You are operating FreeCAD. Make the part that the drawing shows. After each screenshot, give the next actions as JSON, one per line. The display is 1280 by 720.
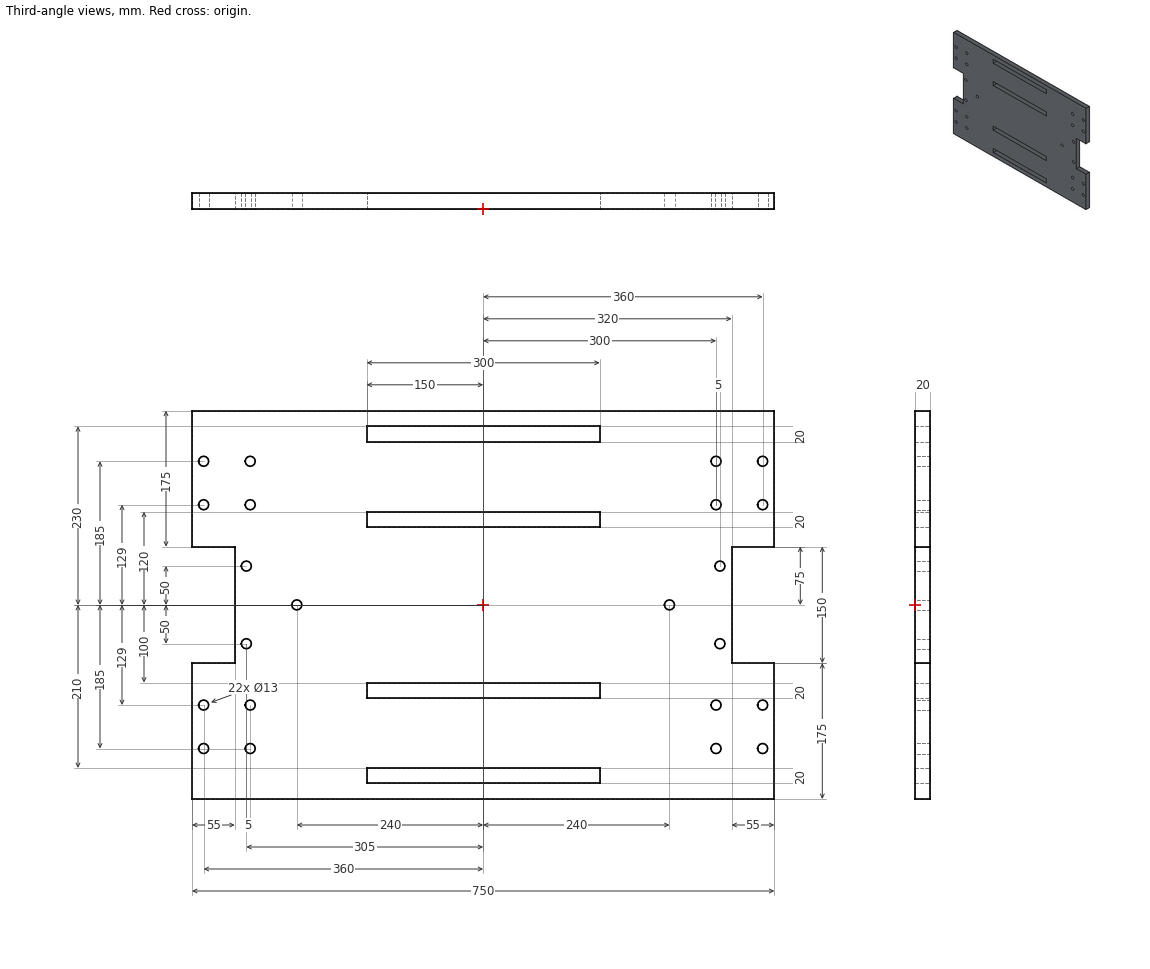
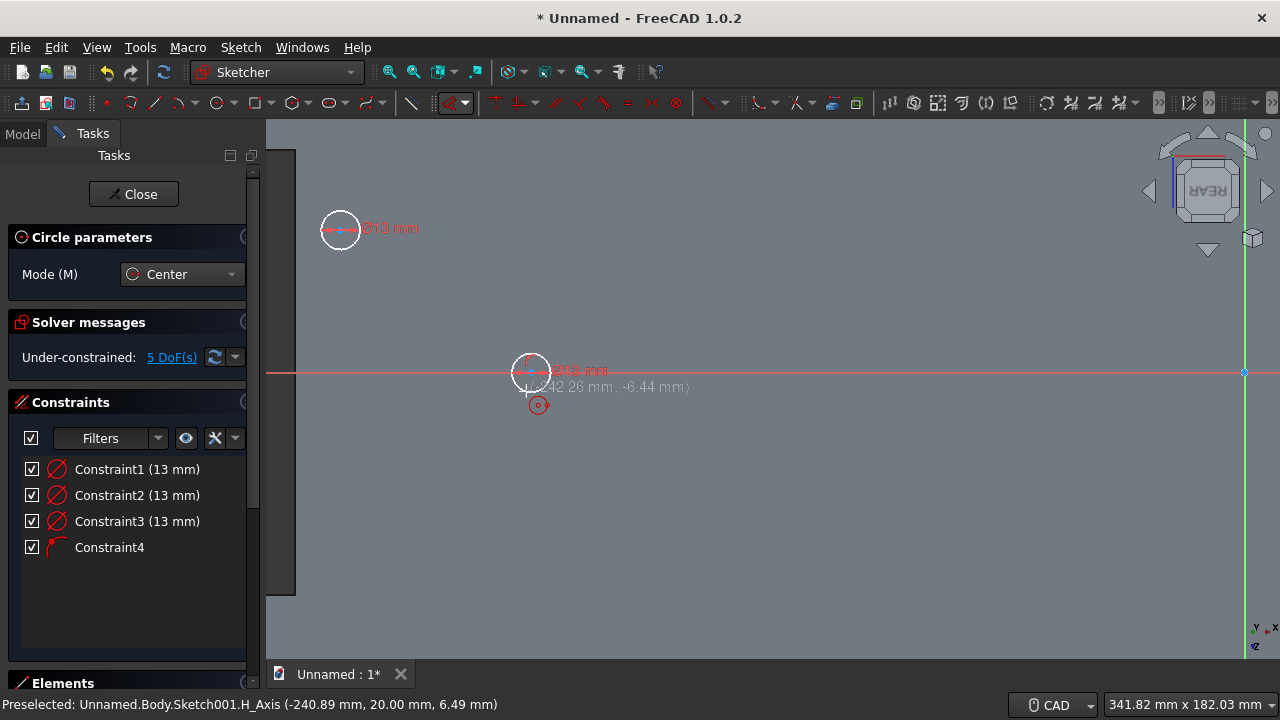
{"action": "scroll", "coordinate": [528, 394], "scroll_direction": "down", "scroll_amount": 7}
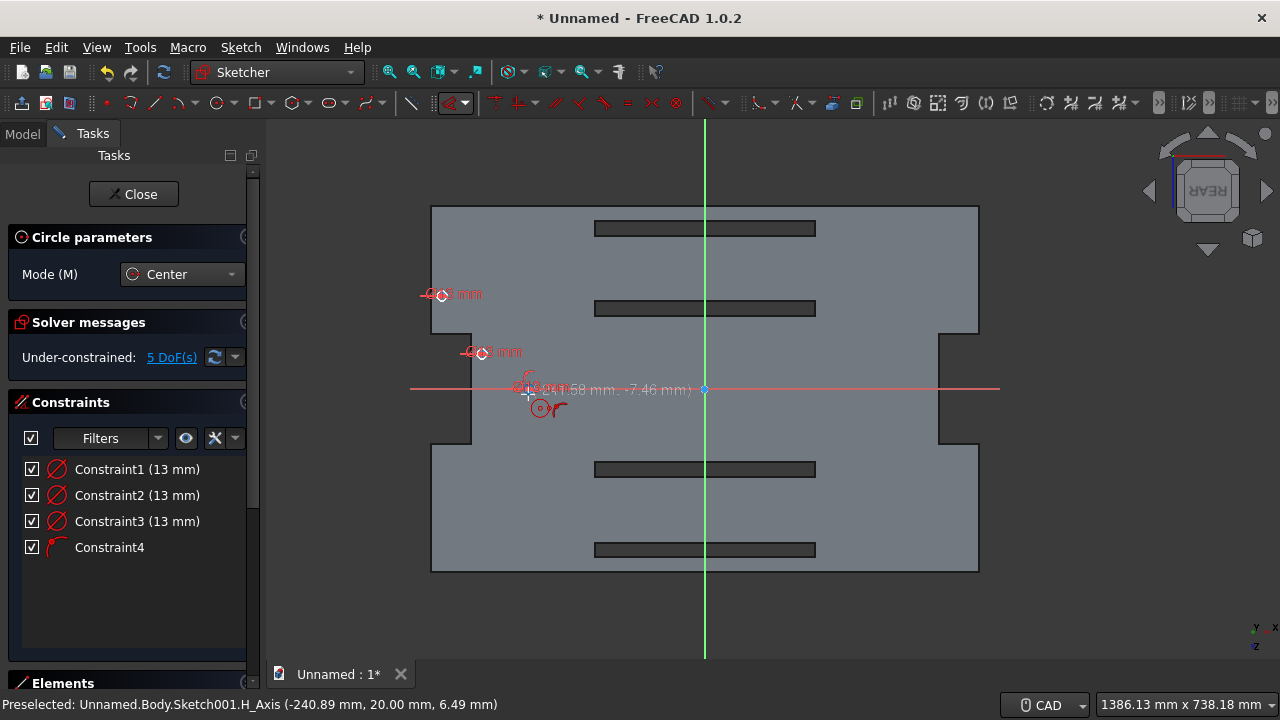
{"action": "scroll", "coordinate": [485, 295], "scroll_direction": "up", "scroll_amount": 8}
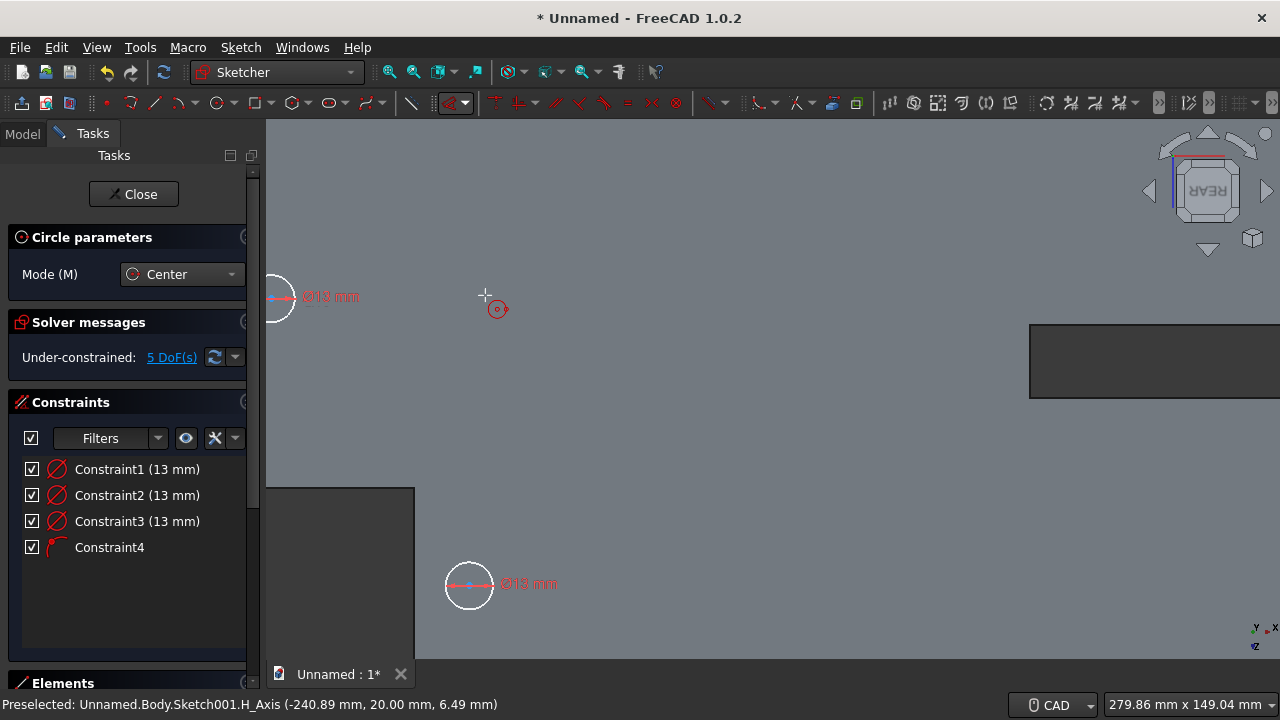
{"action": "scroll", "coordinate": [485, 295], "scroll_direction": "down", "scroll_amount": 8}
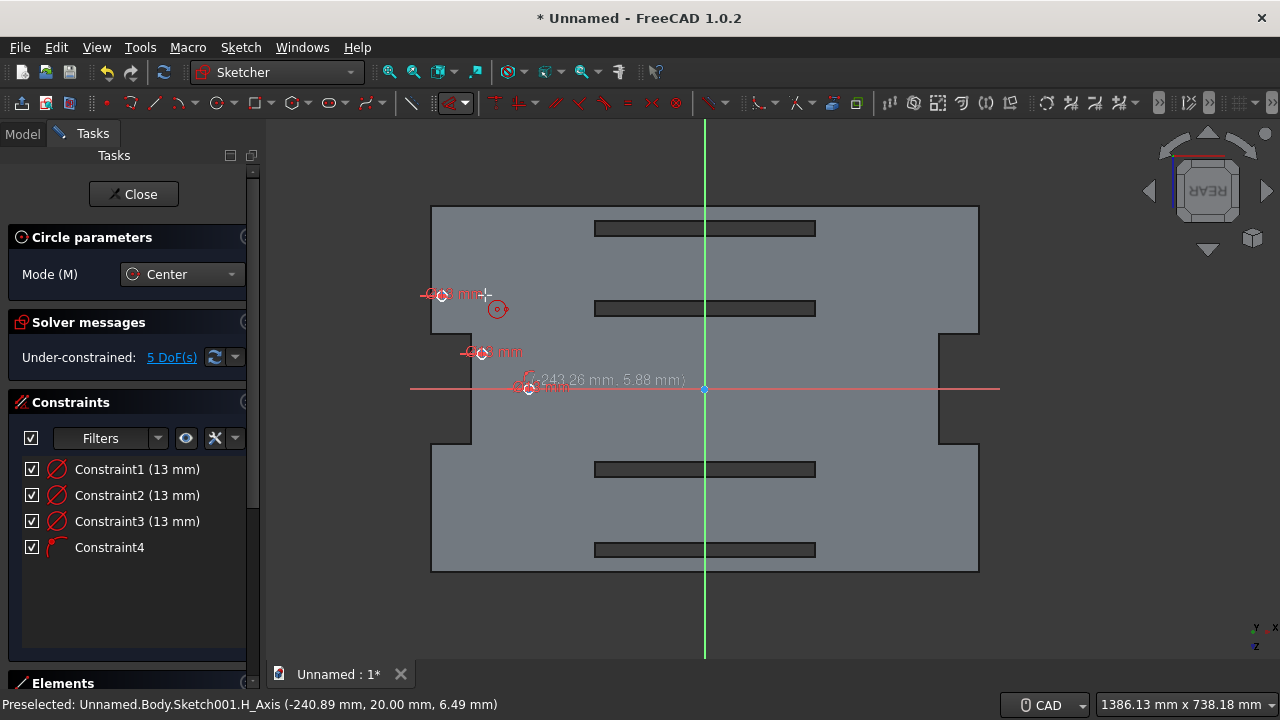
{"action": "left_click", "coordinate": [485, 295]}
{"action": "mouse_move", "coordinate": [489, 291]}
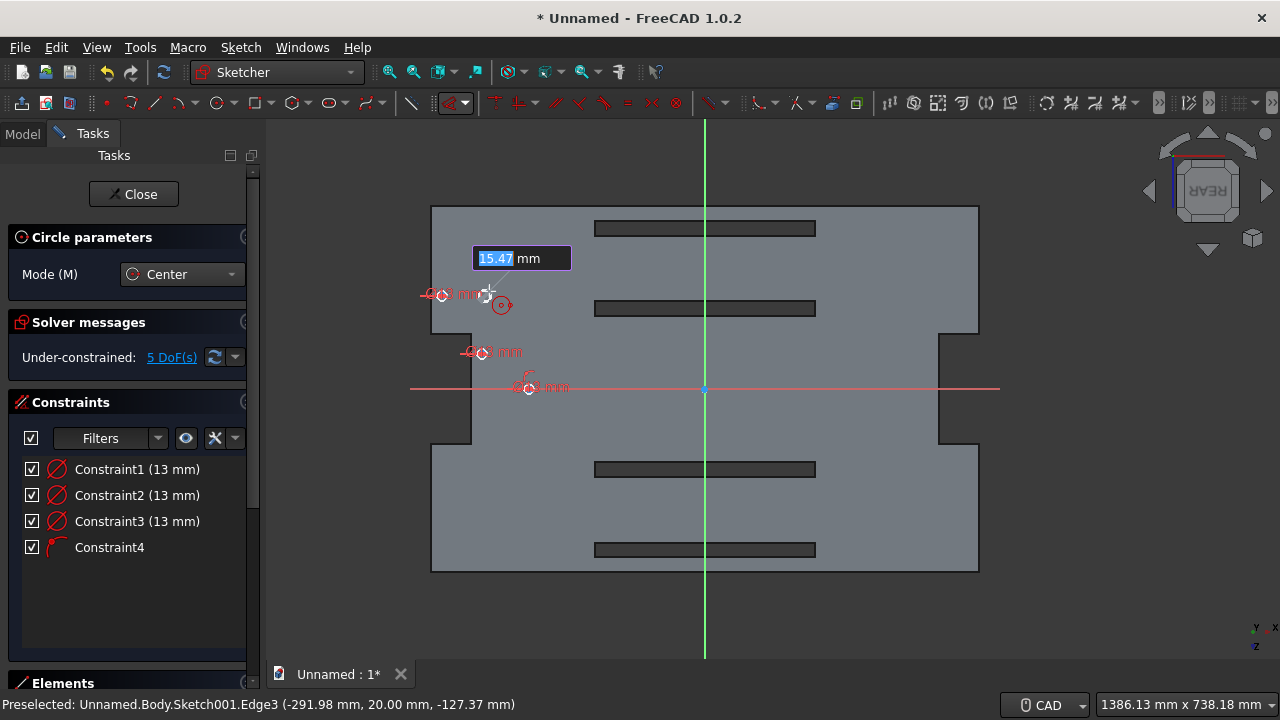
{"action": "type", "text": "13"}
{"action": "key", "text": "Return"}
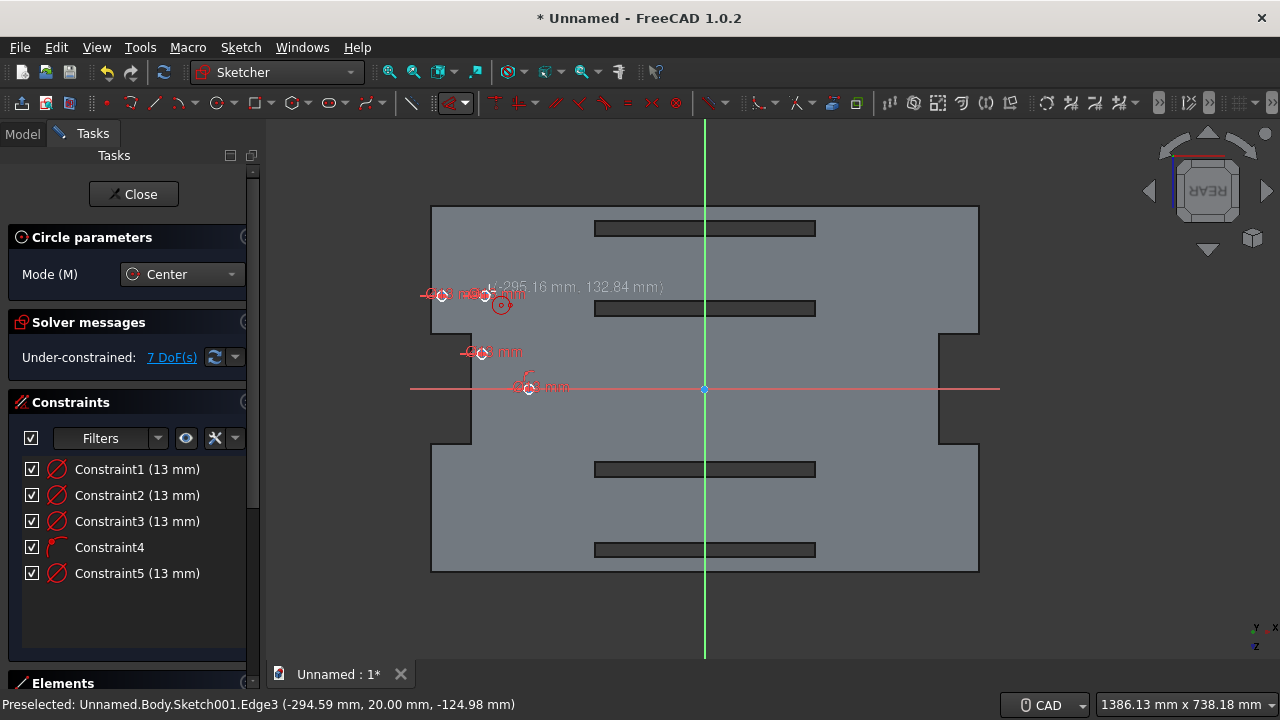
{"action": "scroll", "coordinate": [485, 254], "scroll_direction": "up", "scroll_amount": 8}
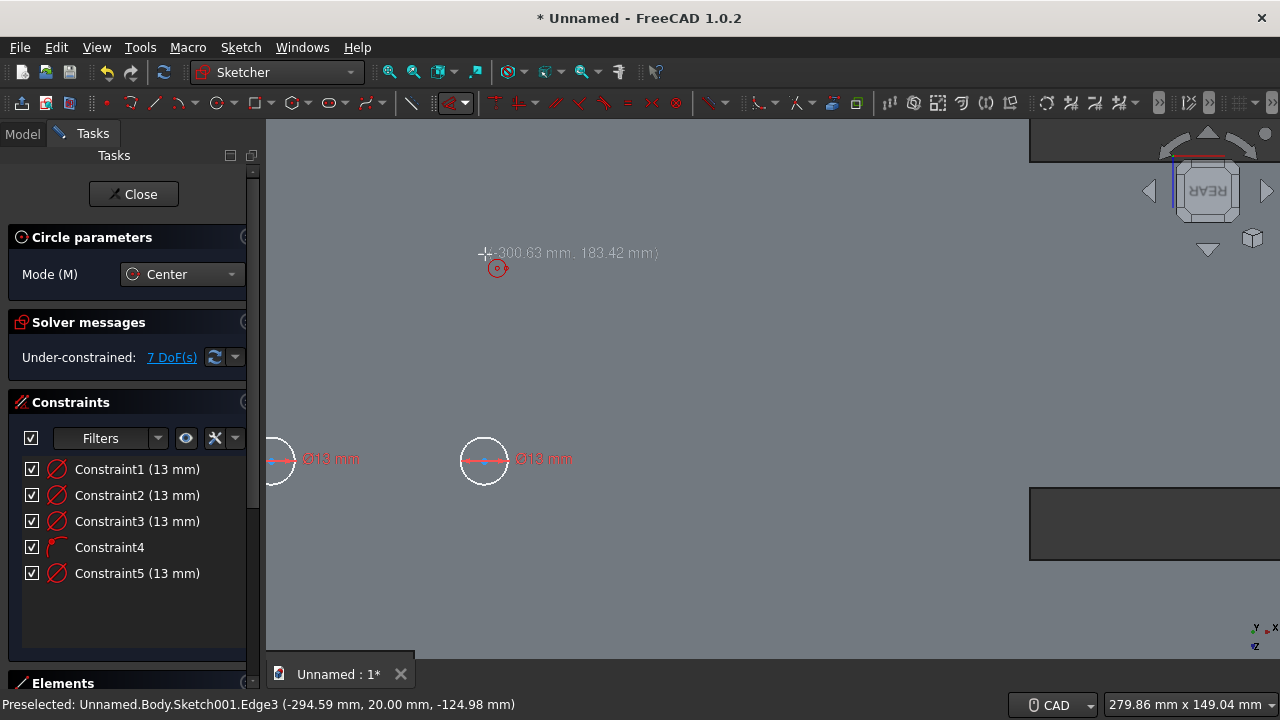
{"action": "scroll", "coordinate": [485, 254], "scroll_direction": "down", "scroll_amount": 8}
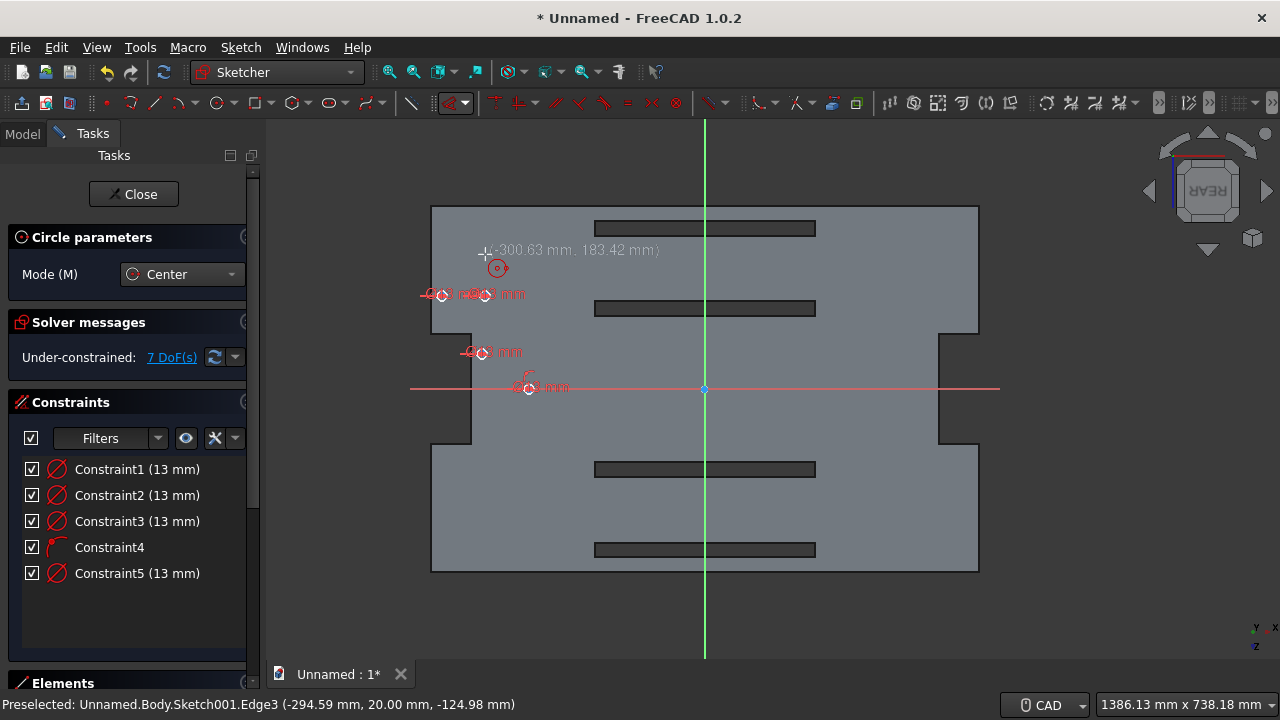
{"action": "left_click", "coordinate": [485, 254]}
{"action": "mouse_move", "coordinate": [489, 250]}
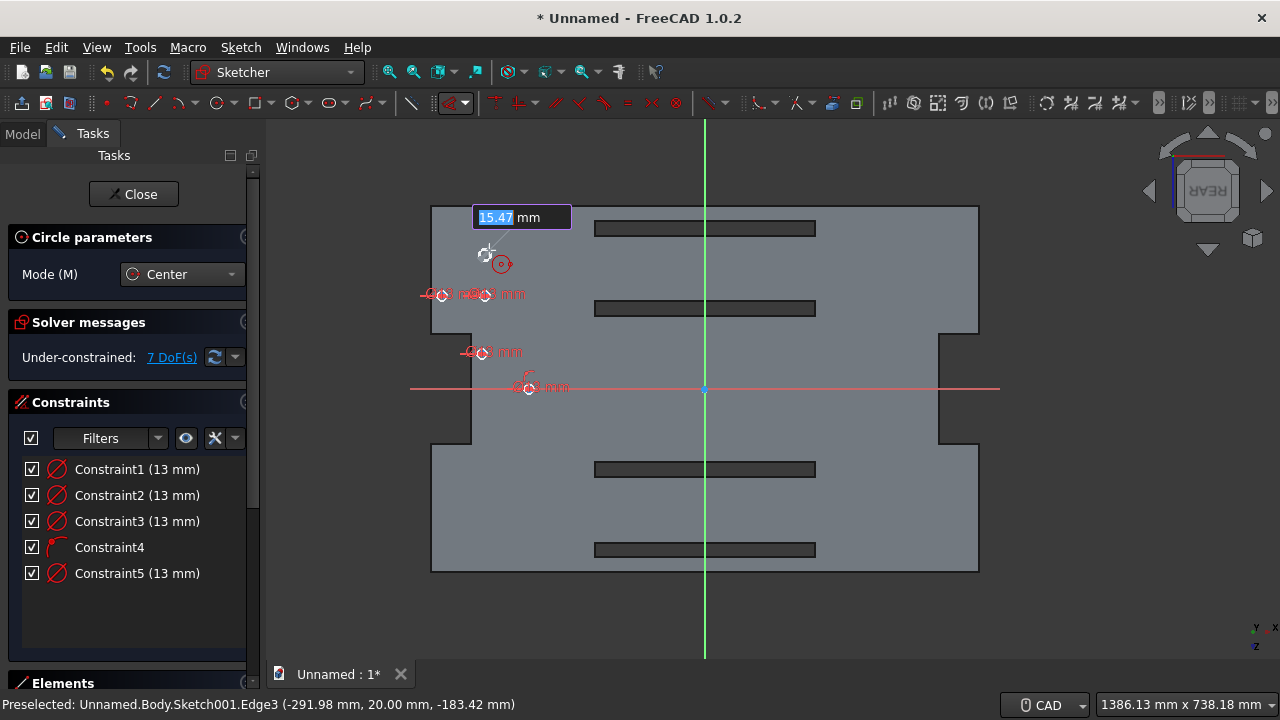
{"action": "type", "text": "13"}
{"action": "key", "text": "Return"}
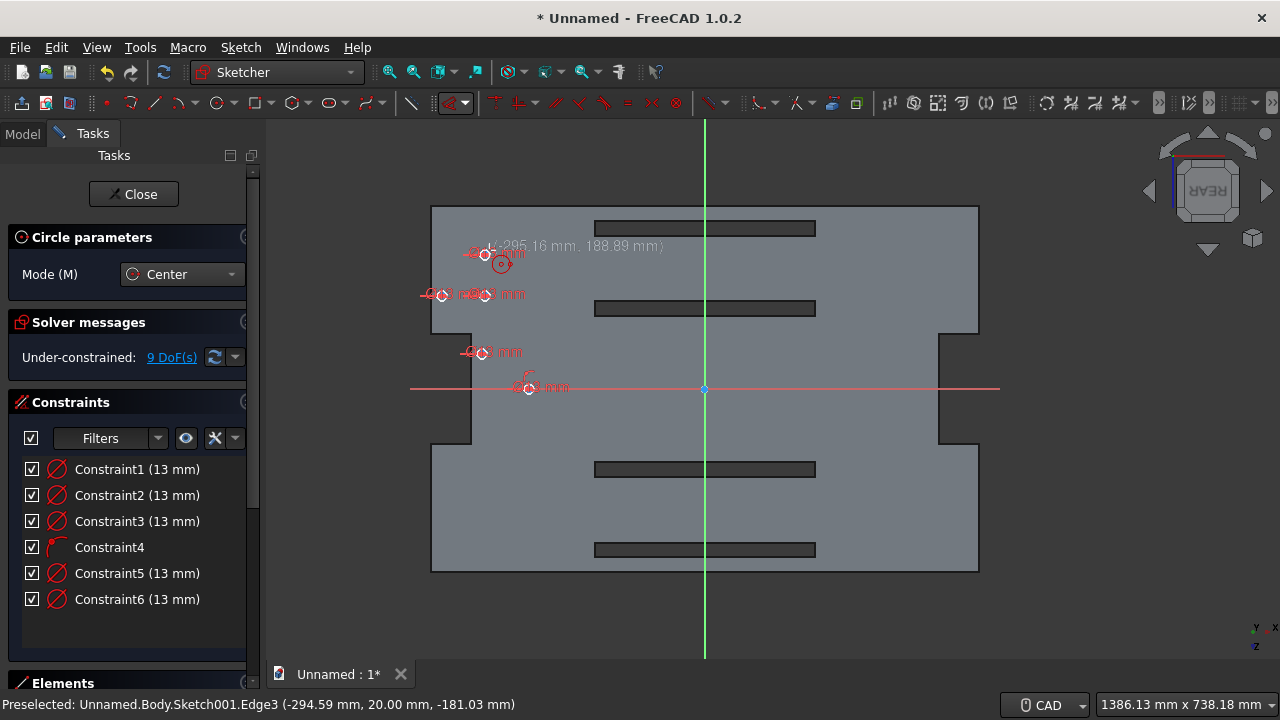
{"action": "scroll", "coordinate": [442, 254], "scroll_direction": "up", "scroll_amount": 8}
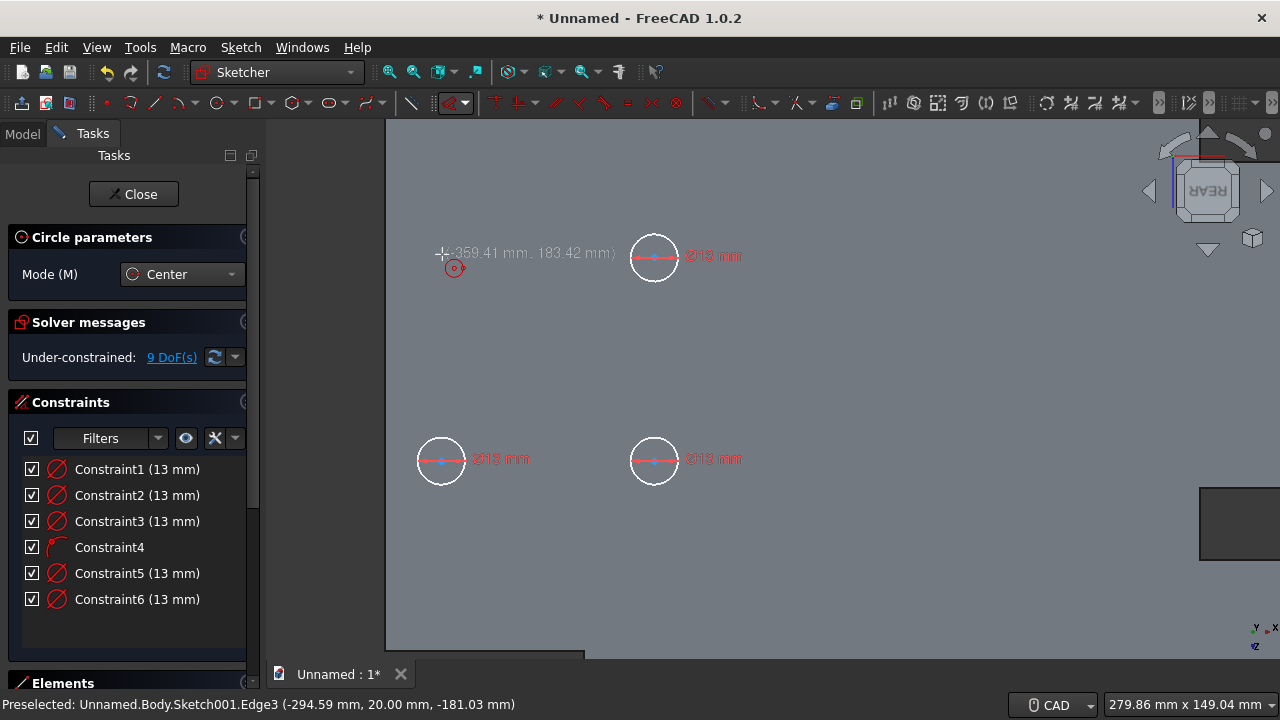
{"action": "scroll", "coordinate": [442, 254], "scroll_direction": "down", "scroll_amount": 8}